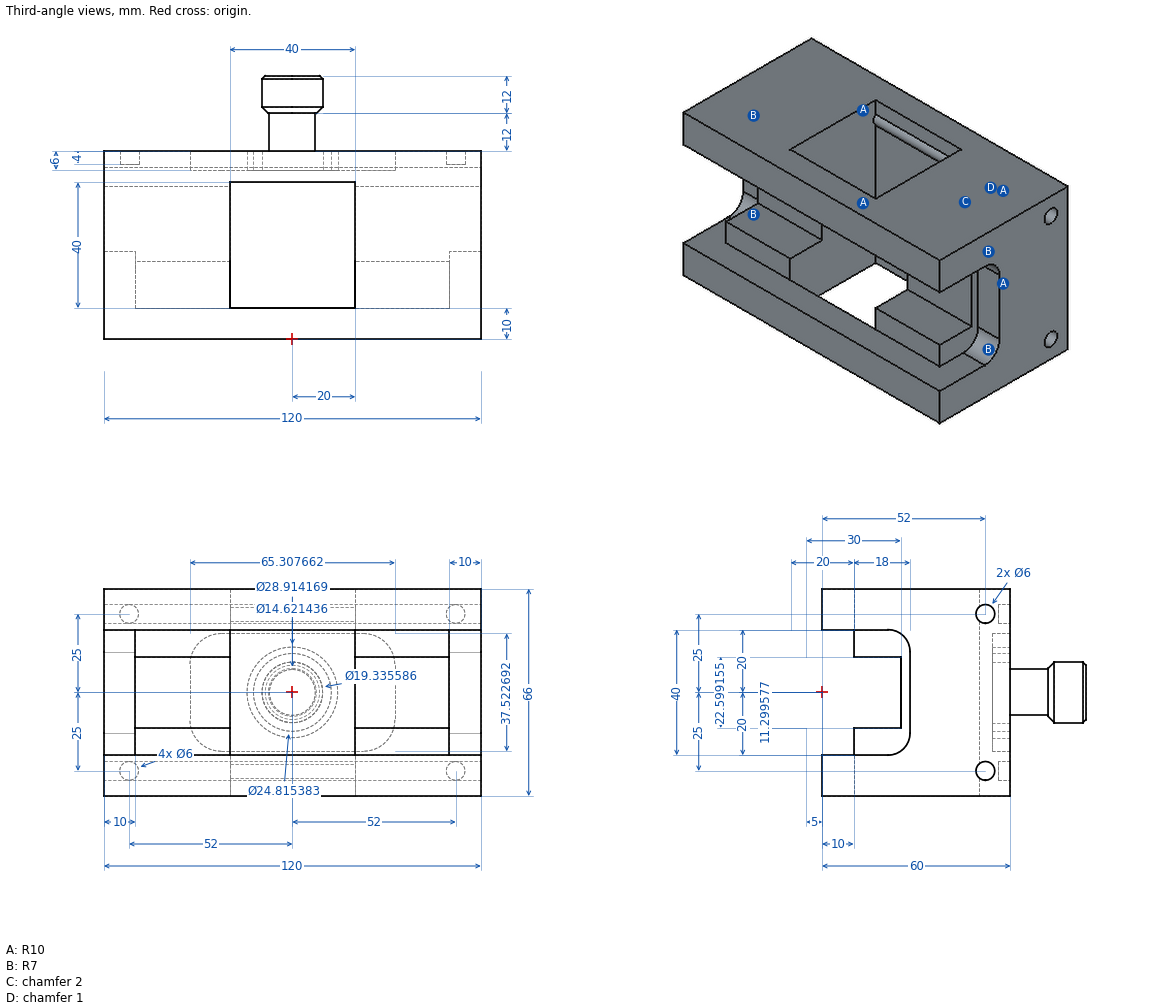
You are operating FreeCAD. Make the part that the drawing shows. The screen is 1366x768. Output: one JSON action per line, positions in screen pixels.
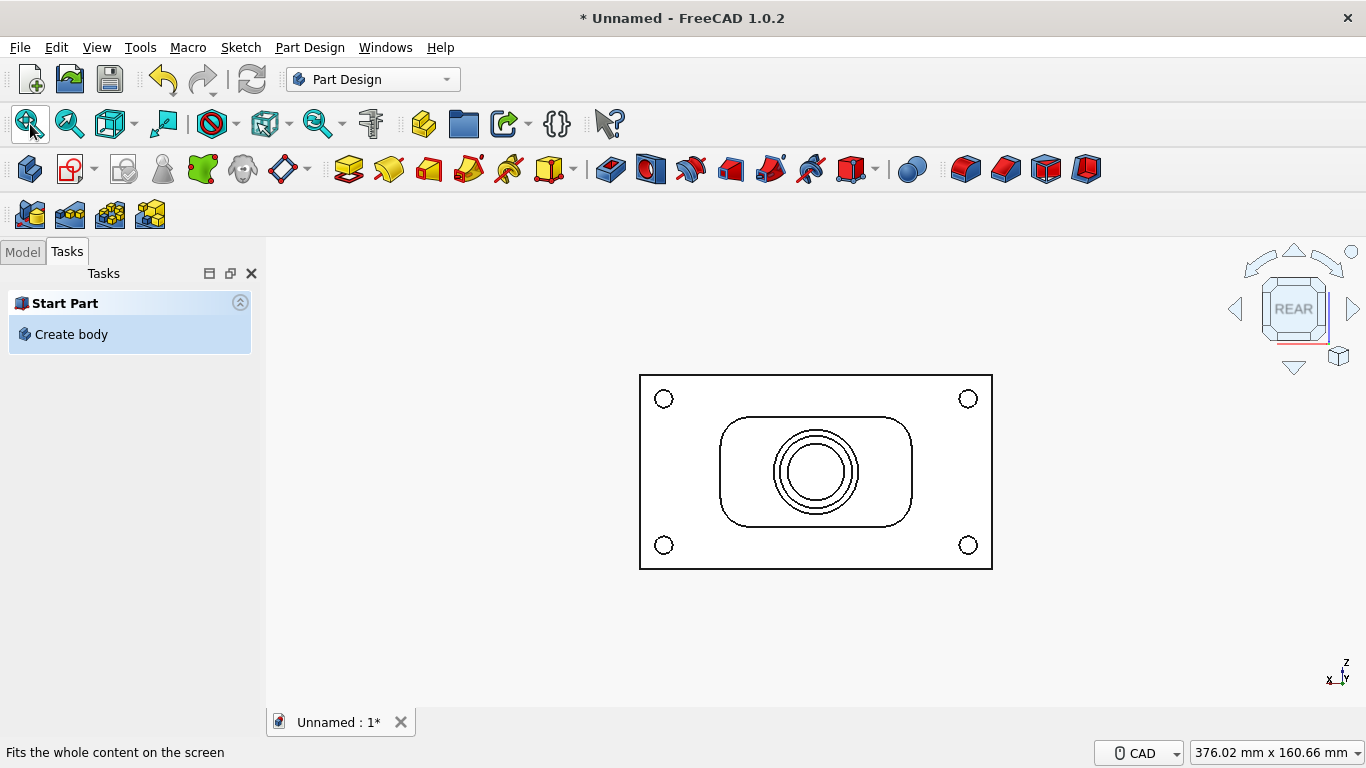
{"action": "key", "text": "0"}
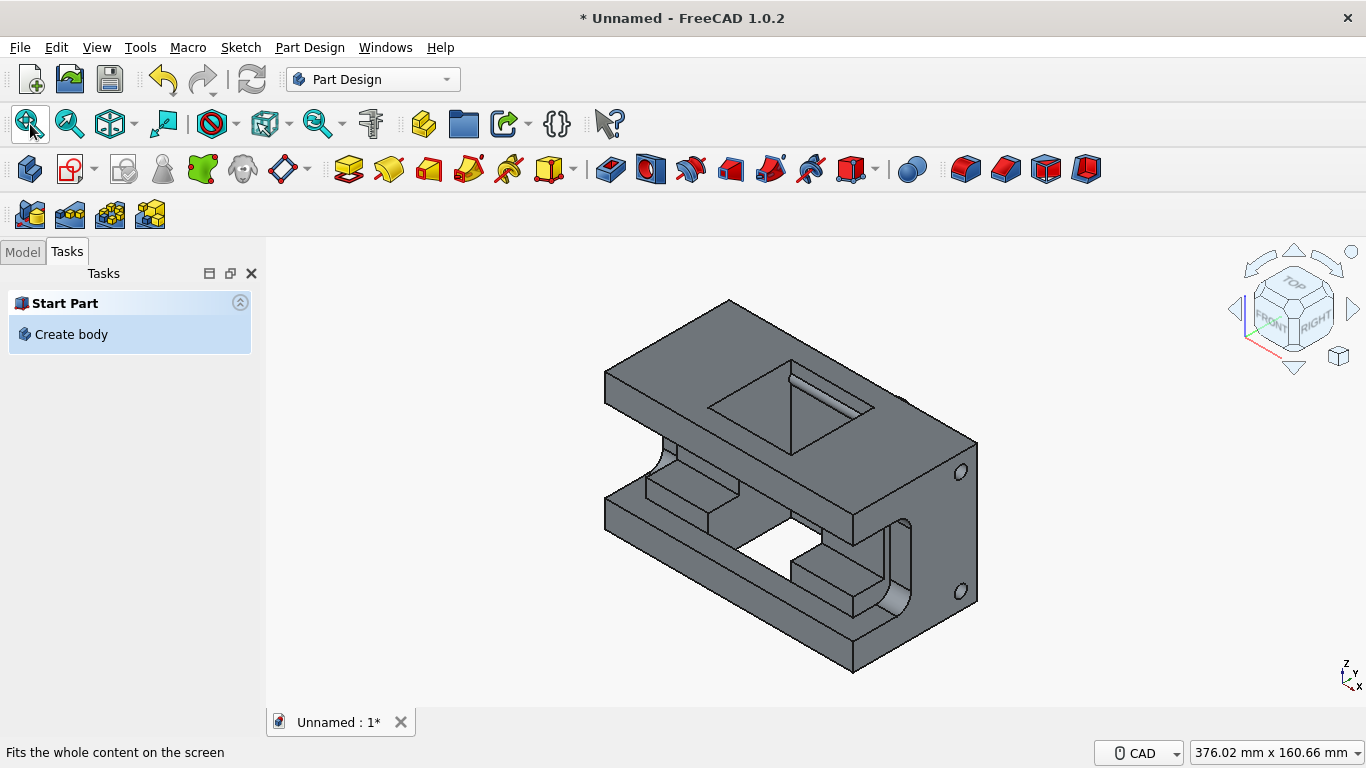
{"action": "key", "text": "2"}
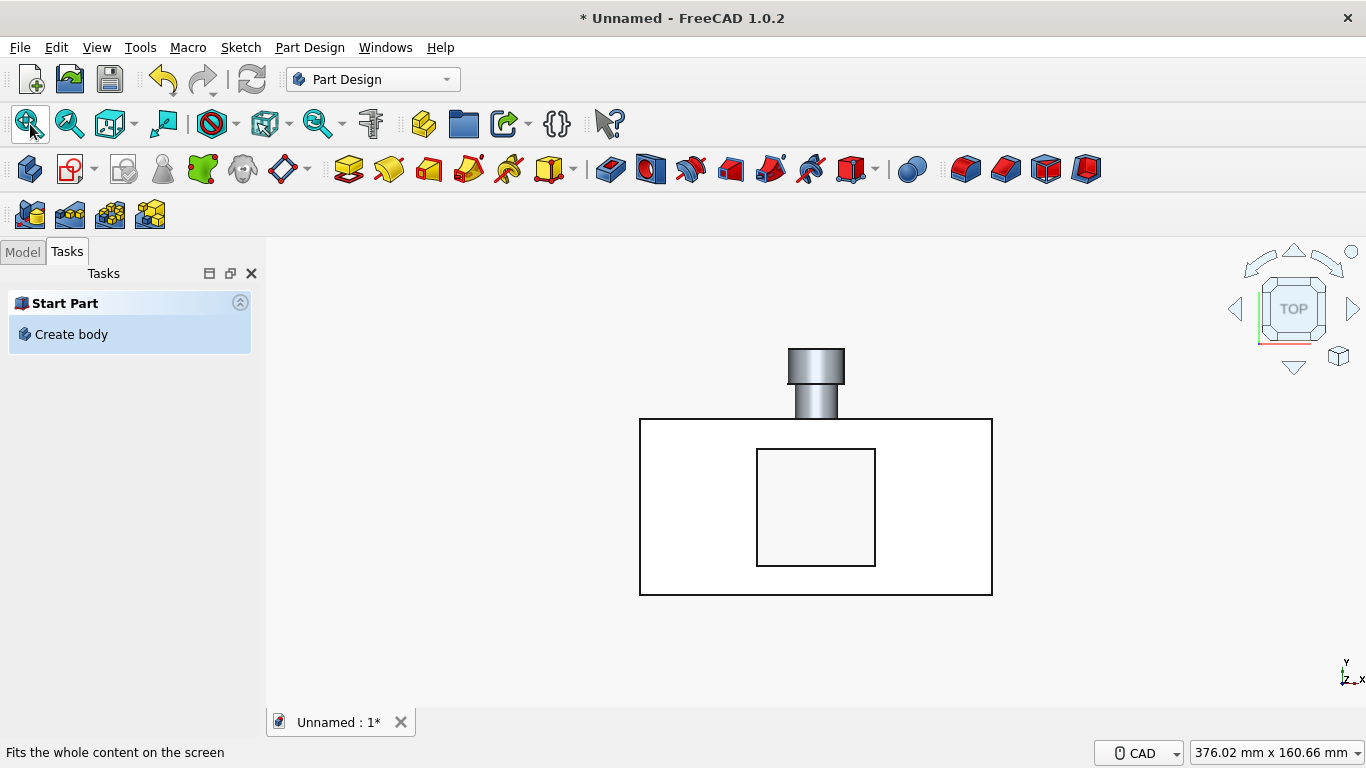
{"action": "left_click", "coordinate": [788, 383]}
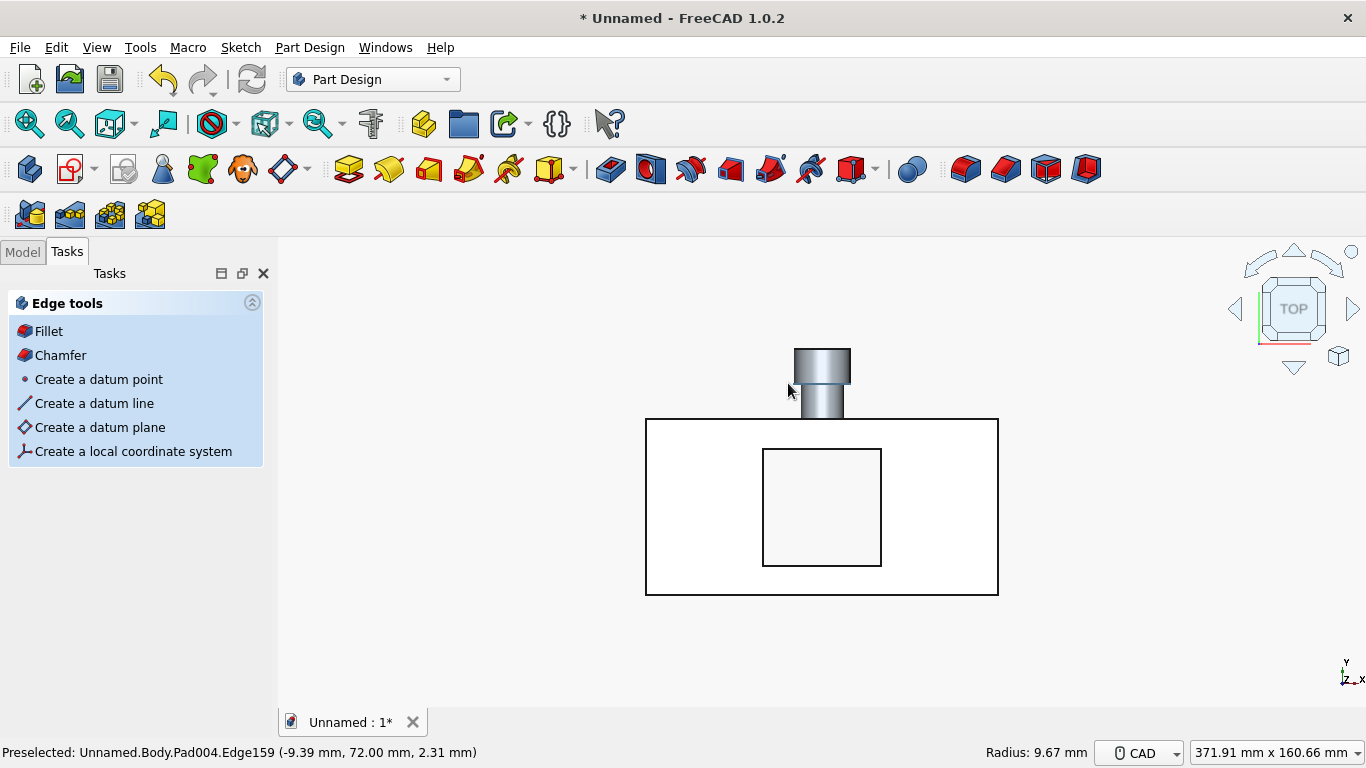
{"action": "left_click", "coordinate": [1006, 170]}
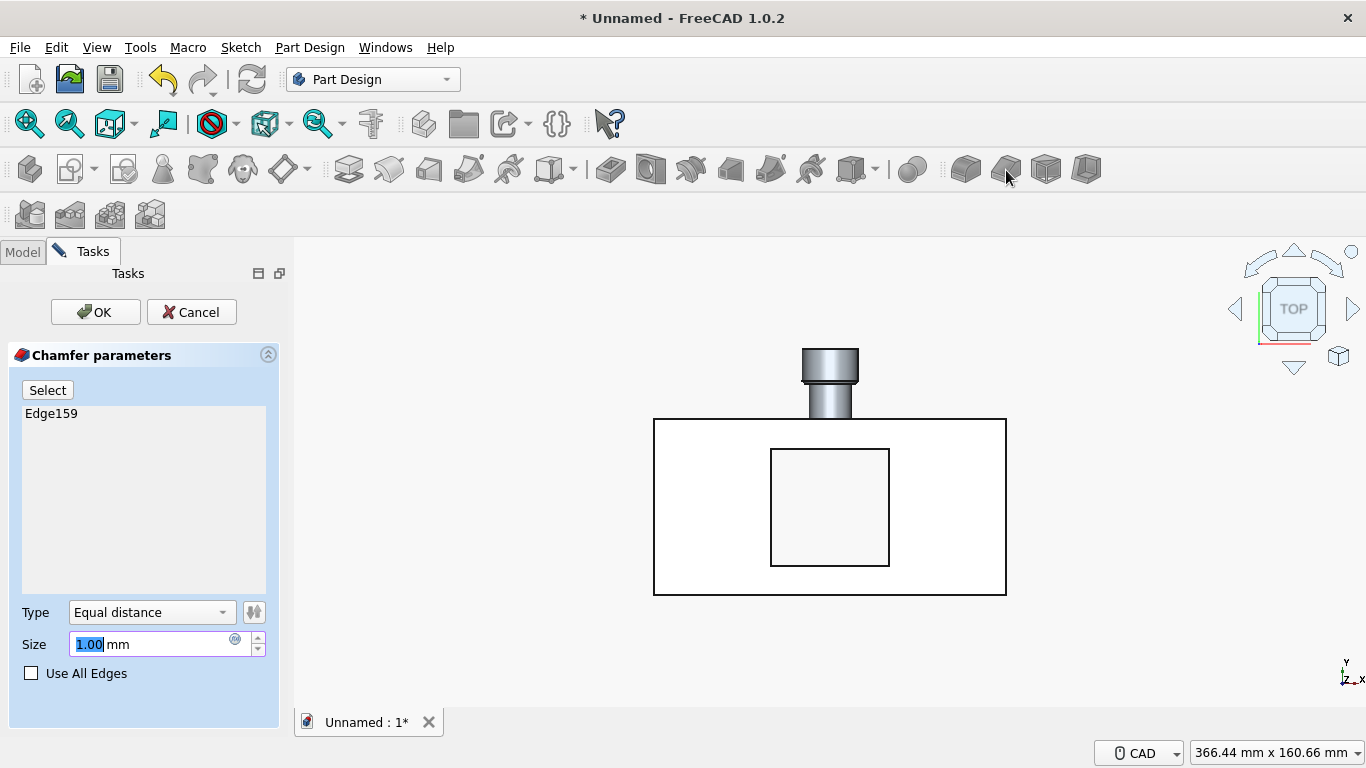
{"action": "type", "text": "2"}
{"action": "key", "text": "Tab"}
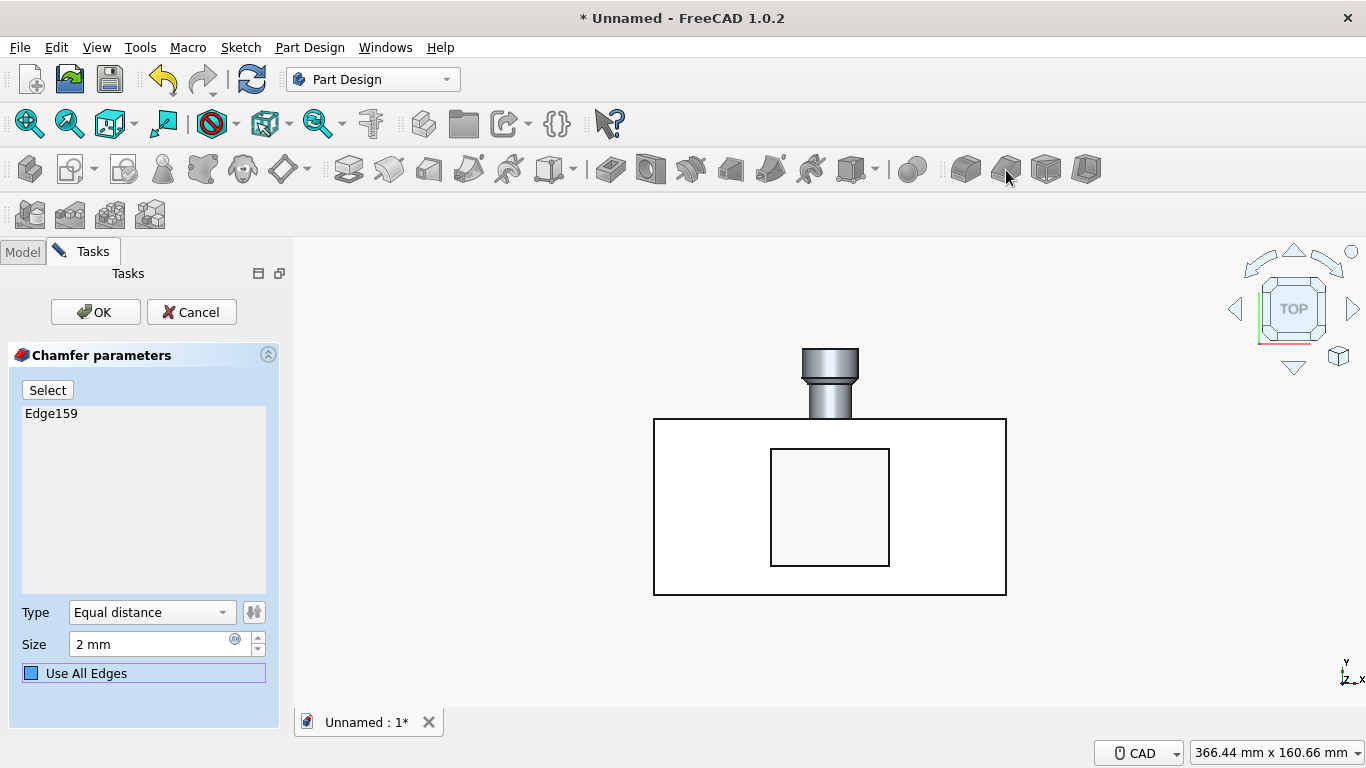
{"action": "left_click", "coordinate": [96, 312]}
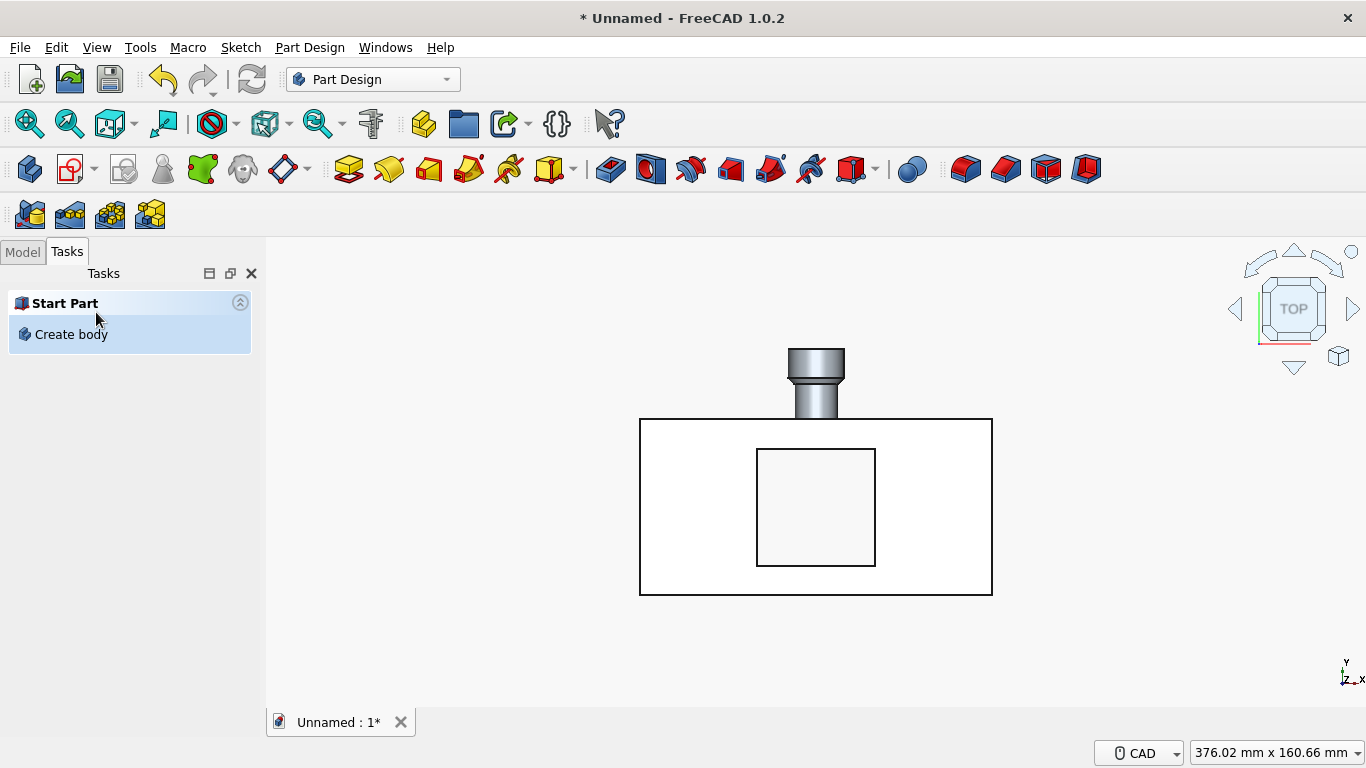
{"action": "left_click", "coordinate": [788, 348]}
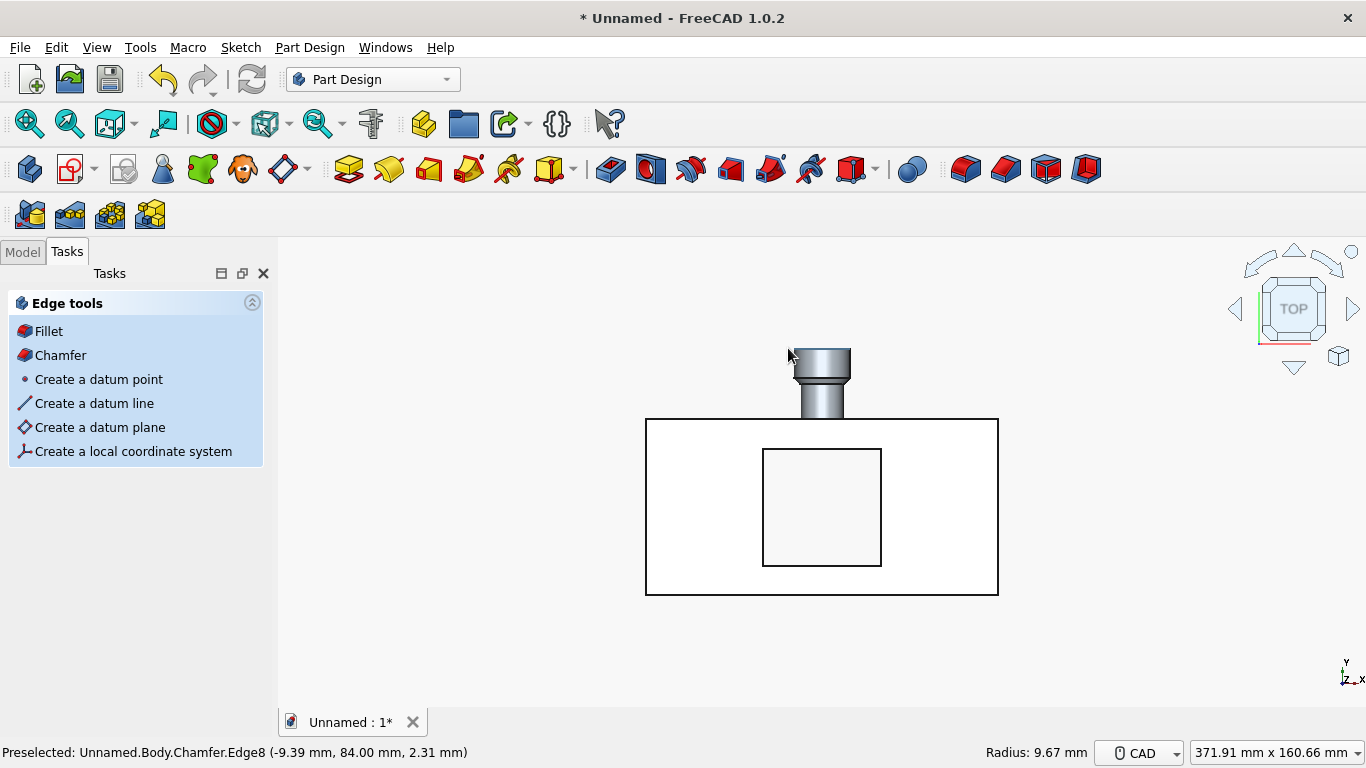
{"action": "left_click", "coordinate": [1006, 170]}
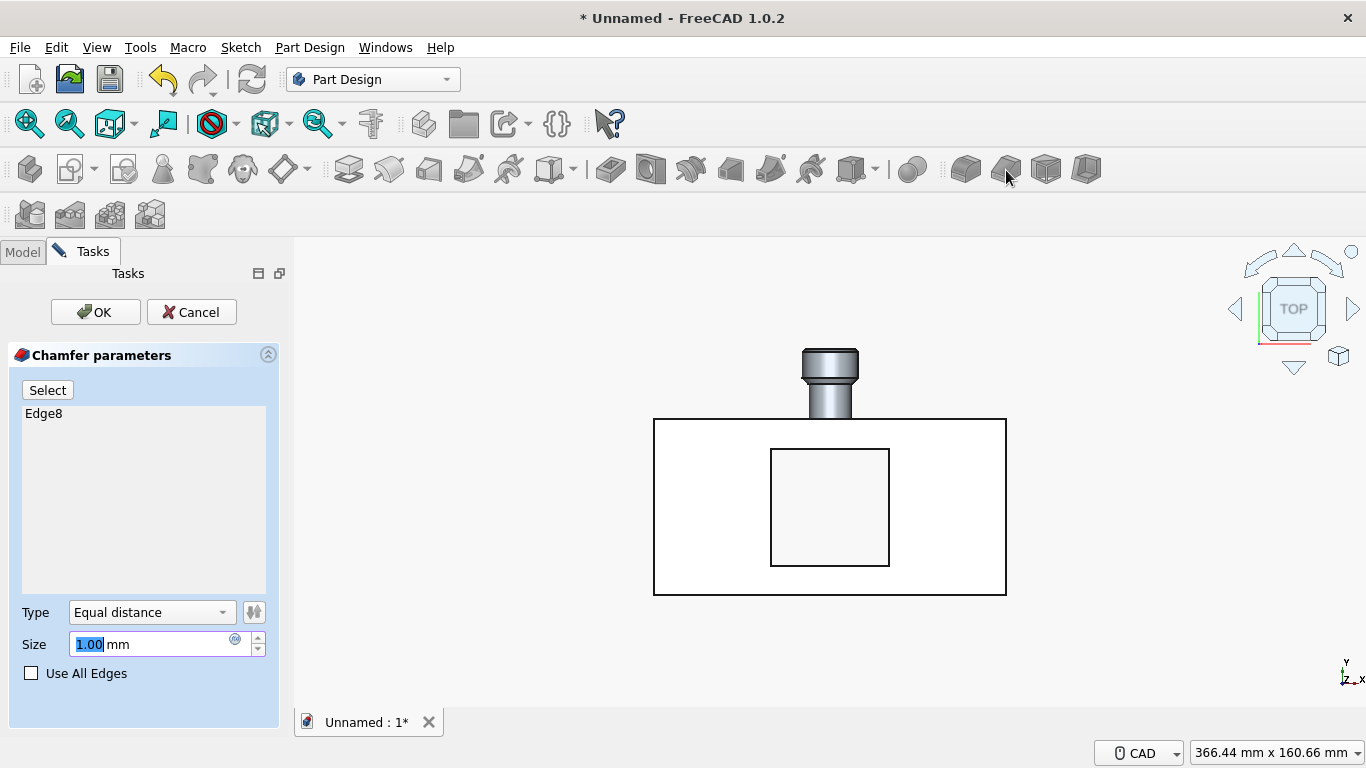
{"action": "type", "text": "1"}
{"action": "key", "text": "Tab"}